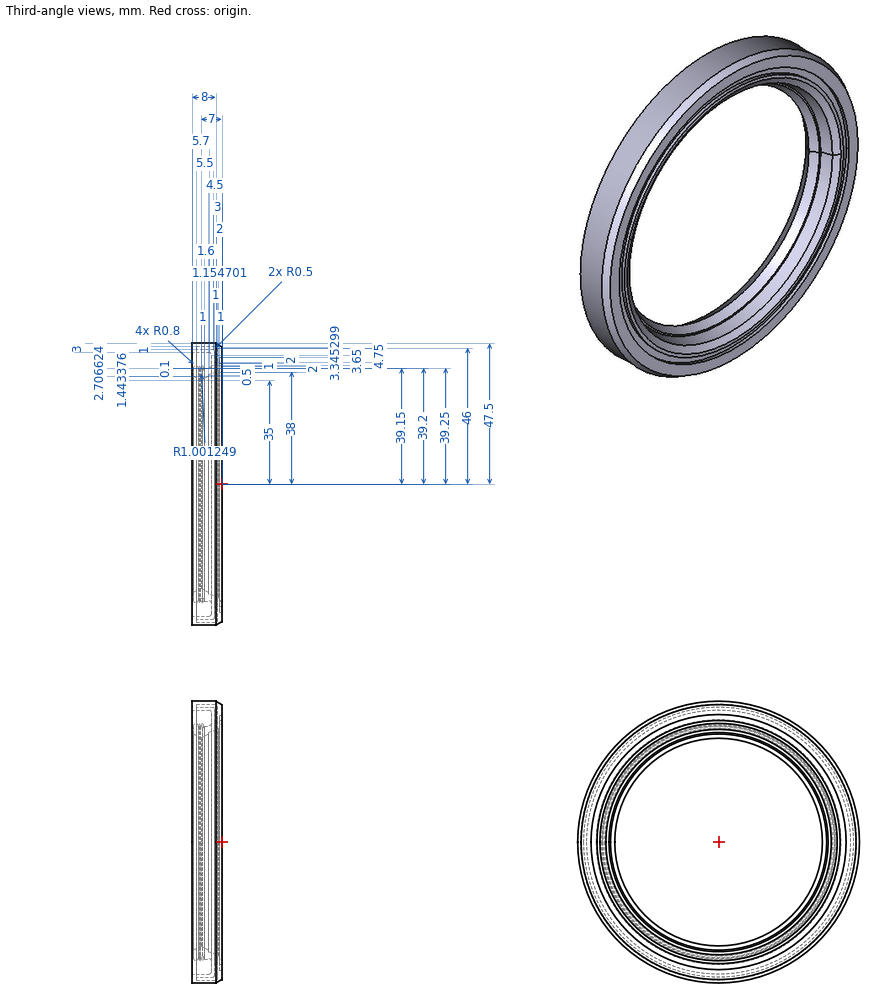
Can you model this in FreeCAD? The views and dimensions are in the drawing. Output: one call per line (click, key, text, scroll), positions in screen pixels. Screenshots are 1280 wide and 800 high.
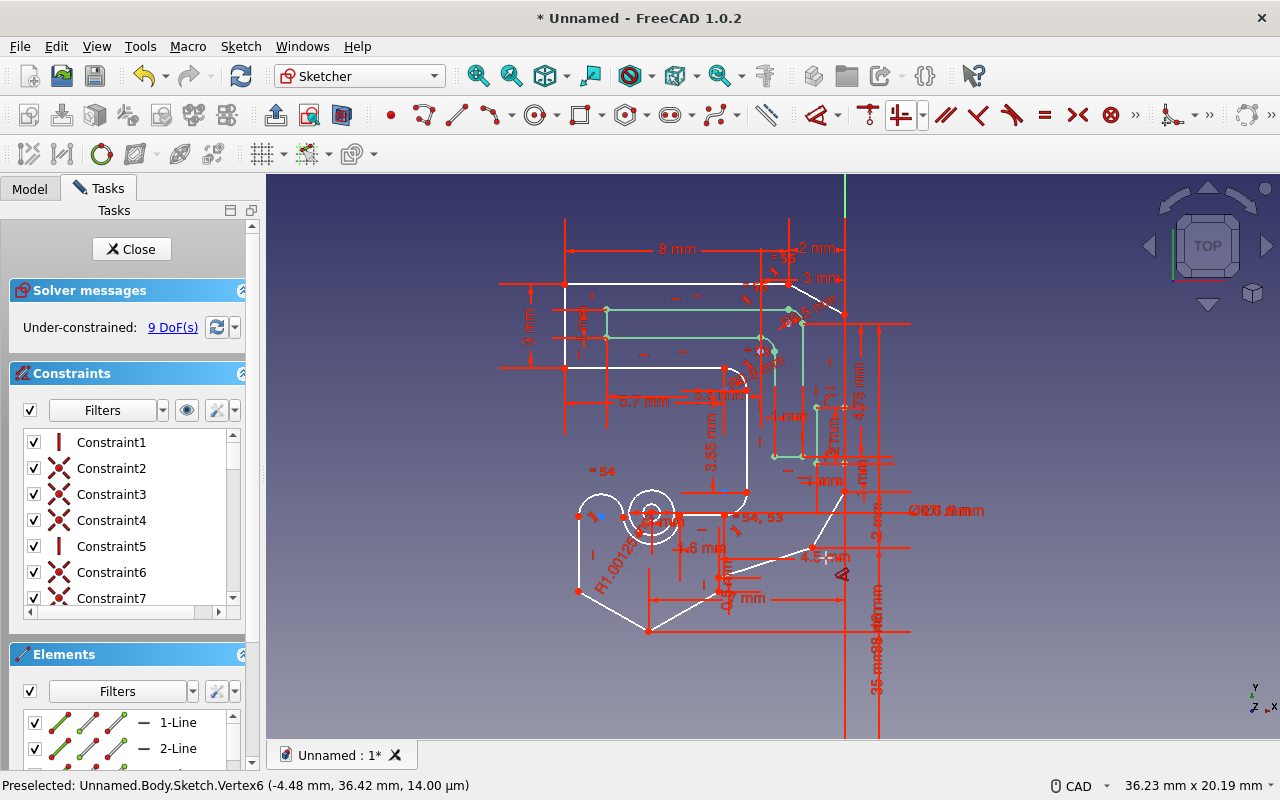
scroll(624, 517, up, 14)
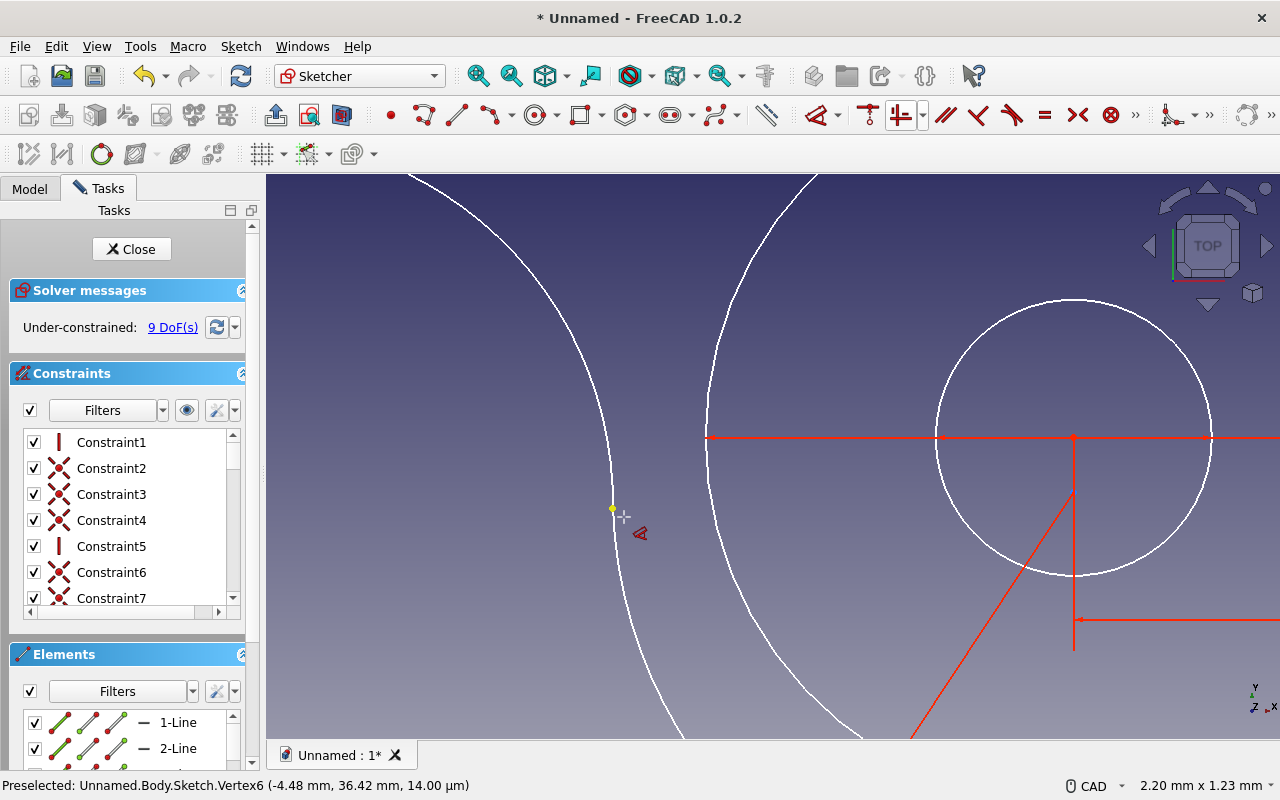
click(613, 508)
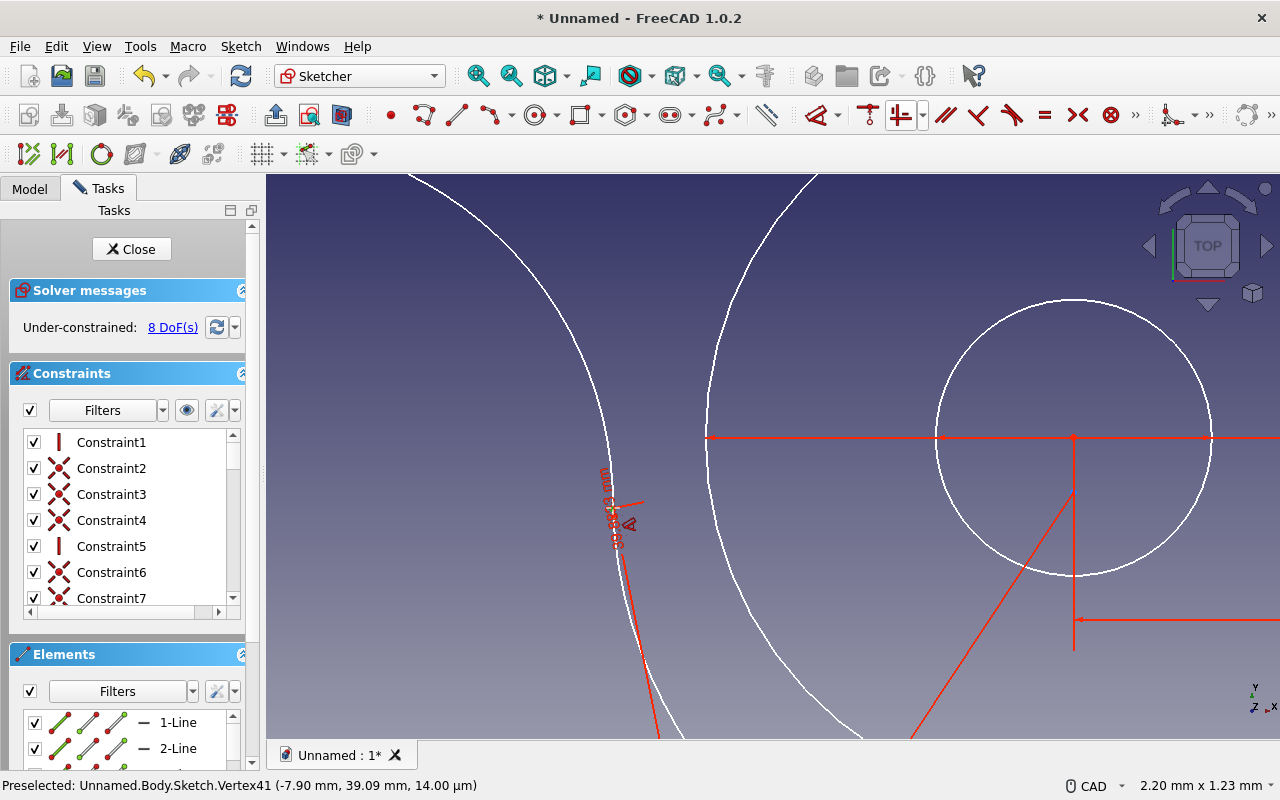
click(1074, 438)
click(579, 473)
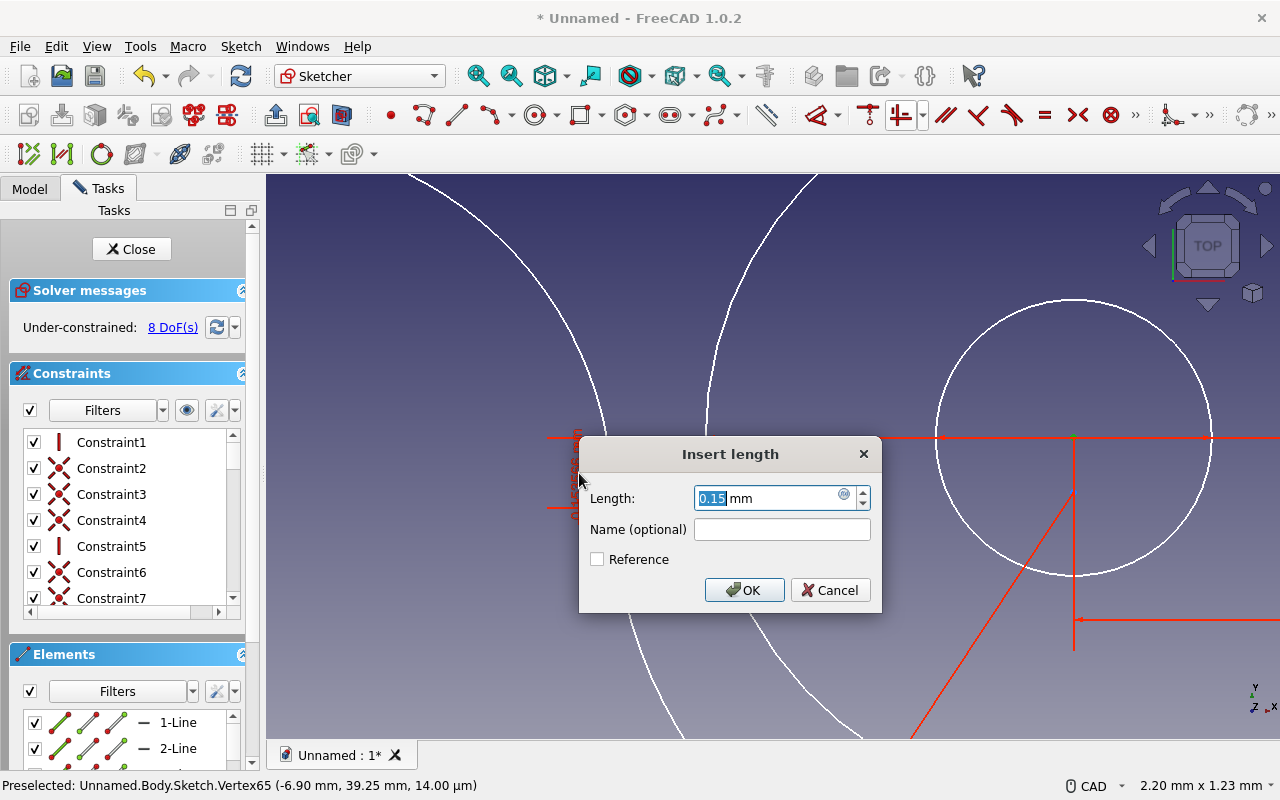
text(0.1)
key(Return)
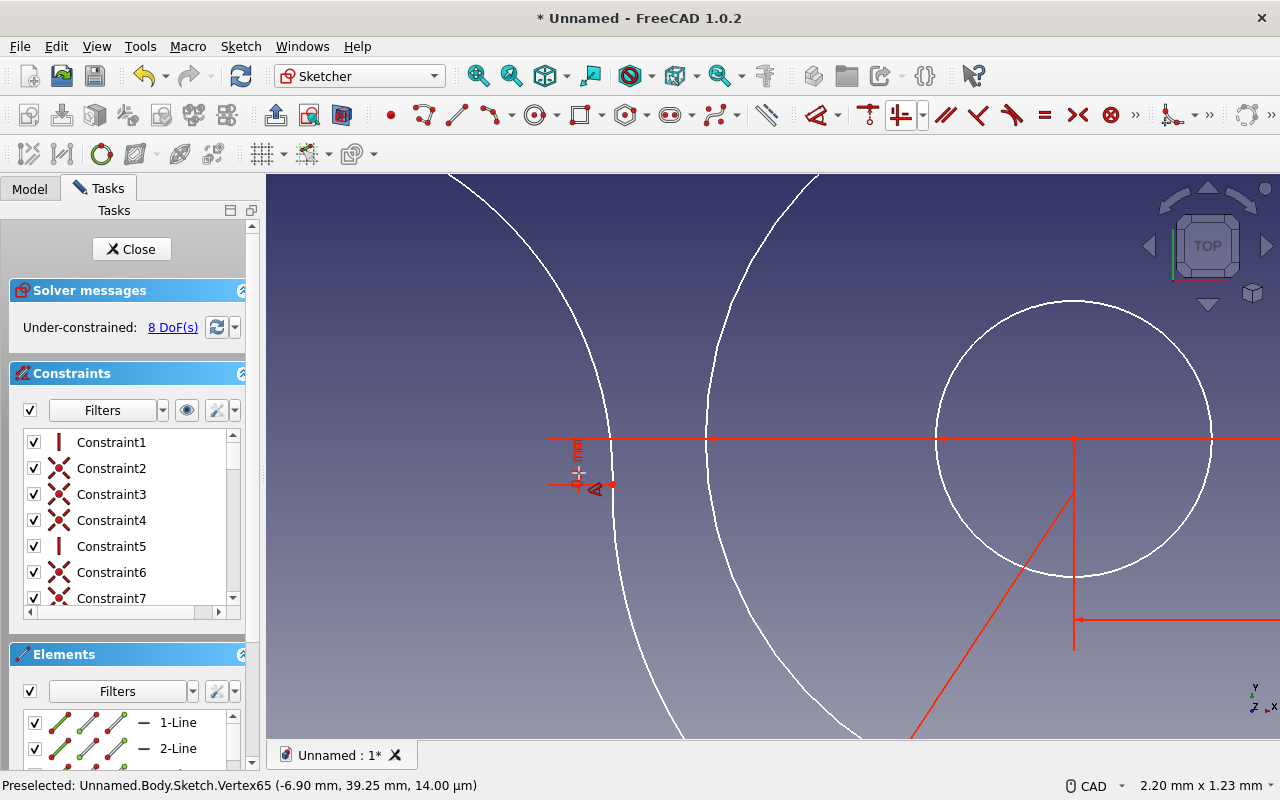
scroll(624, 517, down, 14)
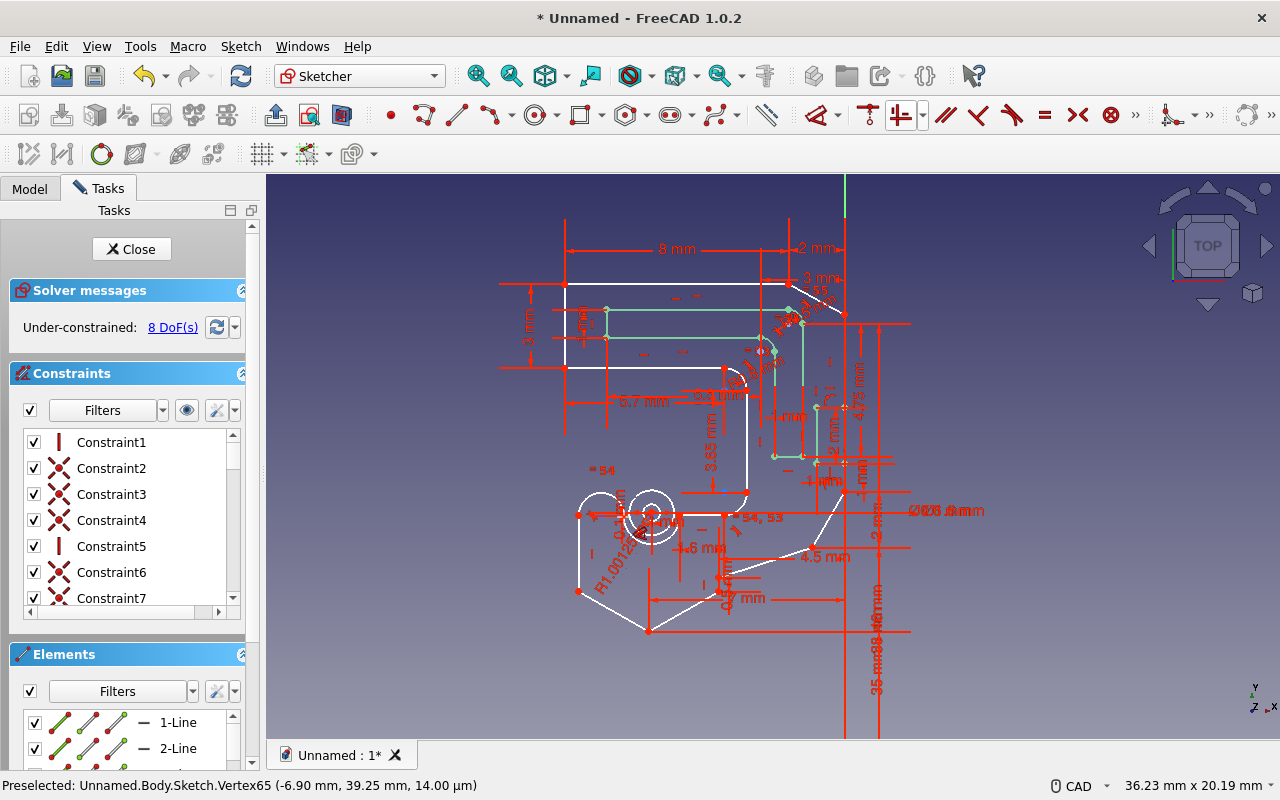
click(789, 284)
click(879, 348)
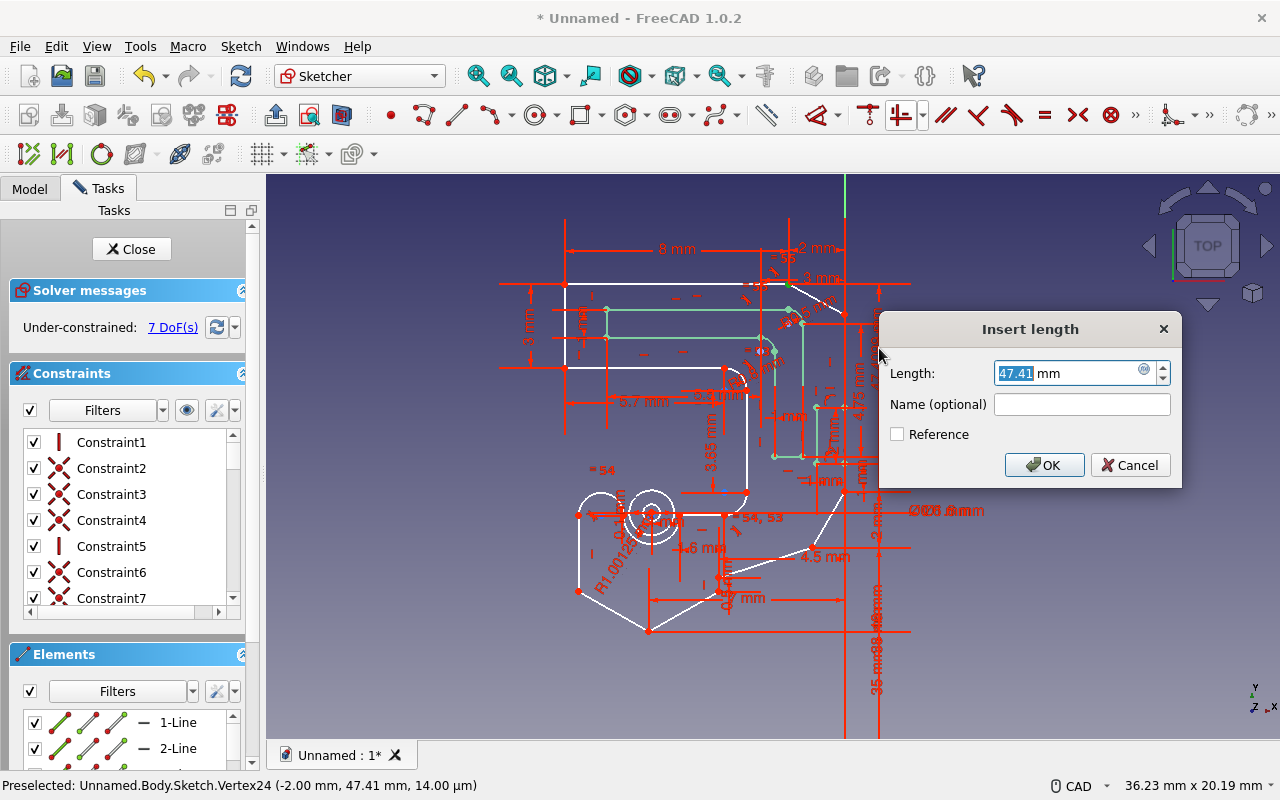
text(47.5)
key(Return)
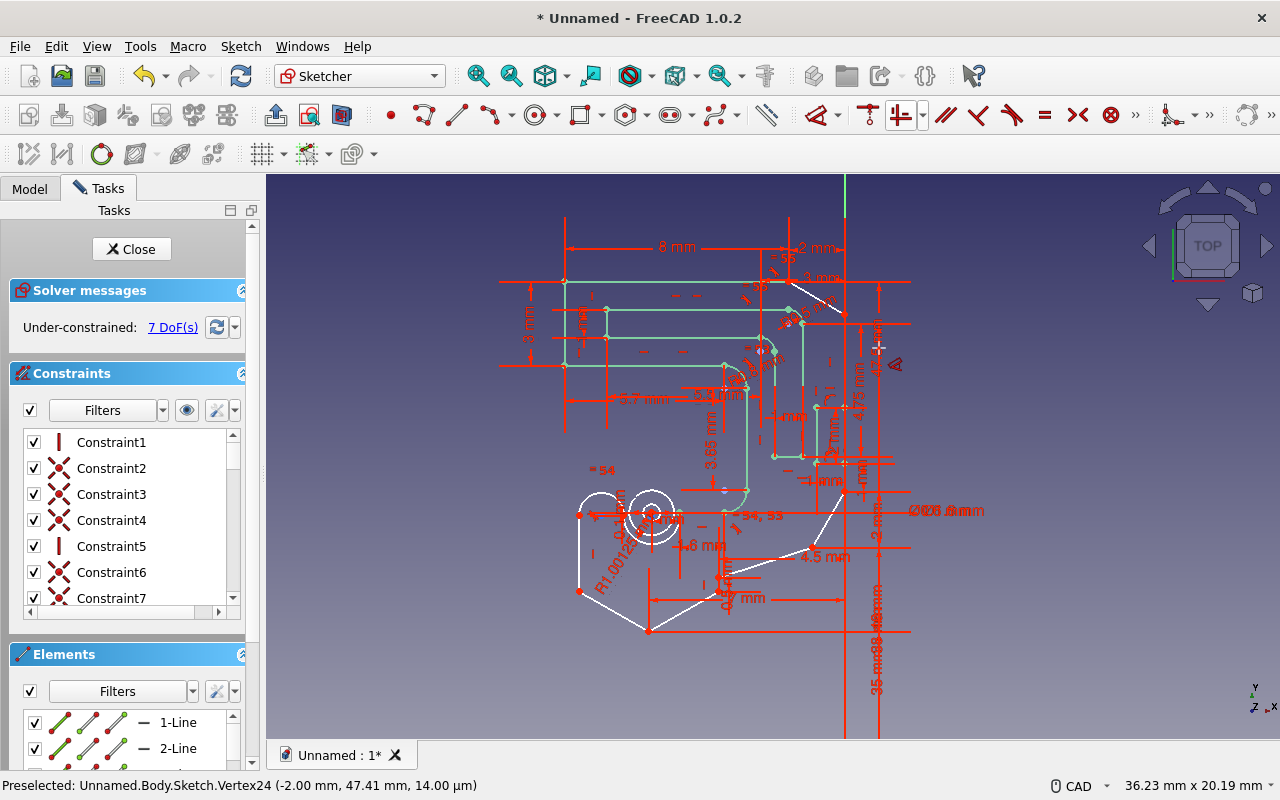
scroll(652, 516, up, 7)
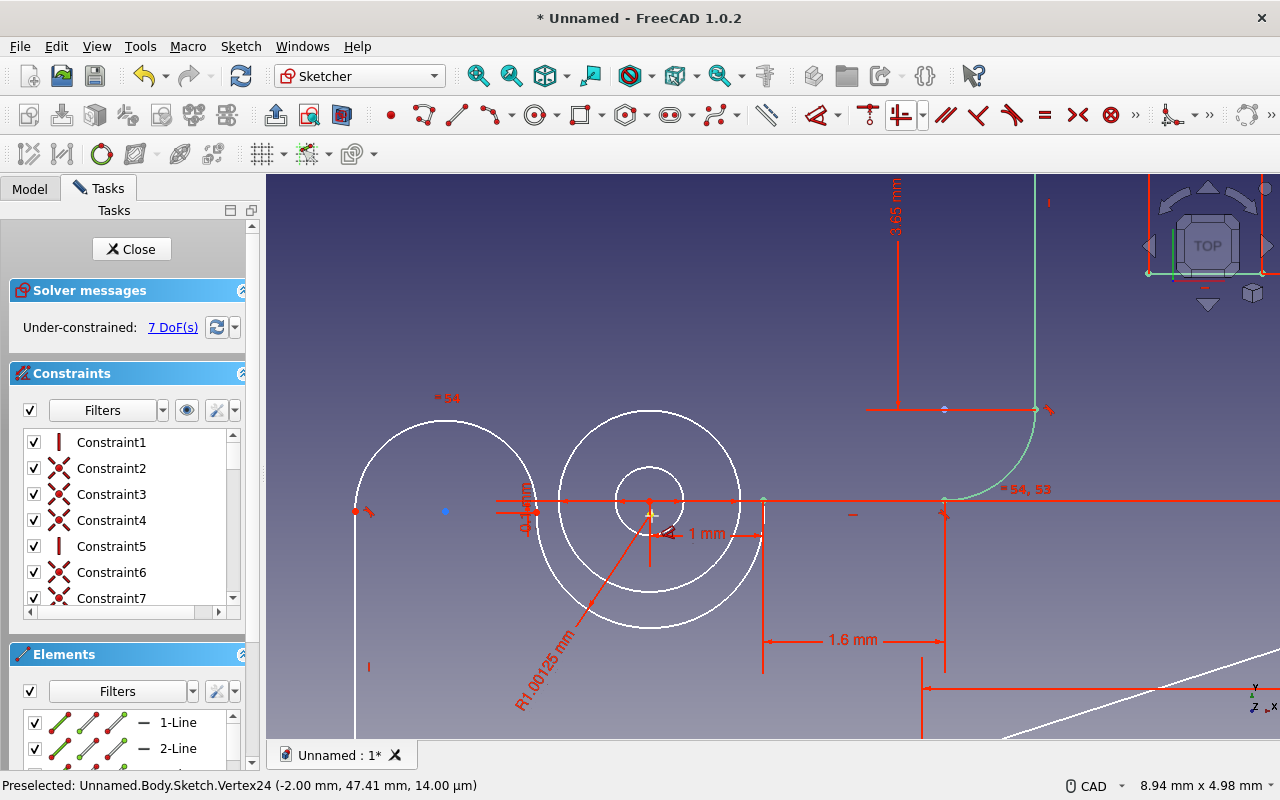
click(650, 514)
click(616, 568)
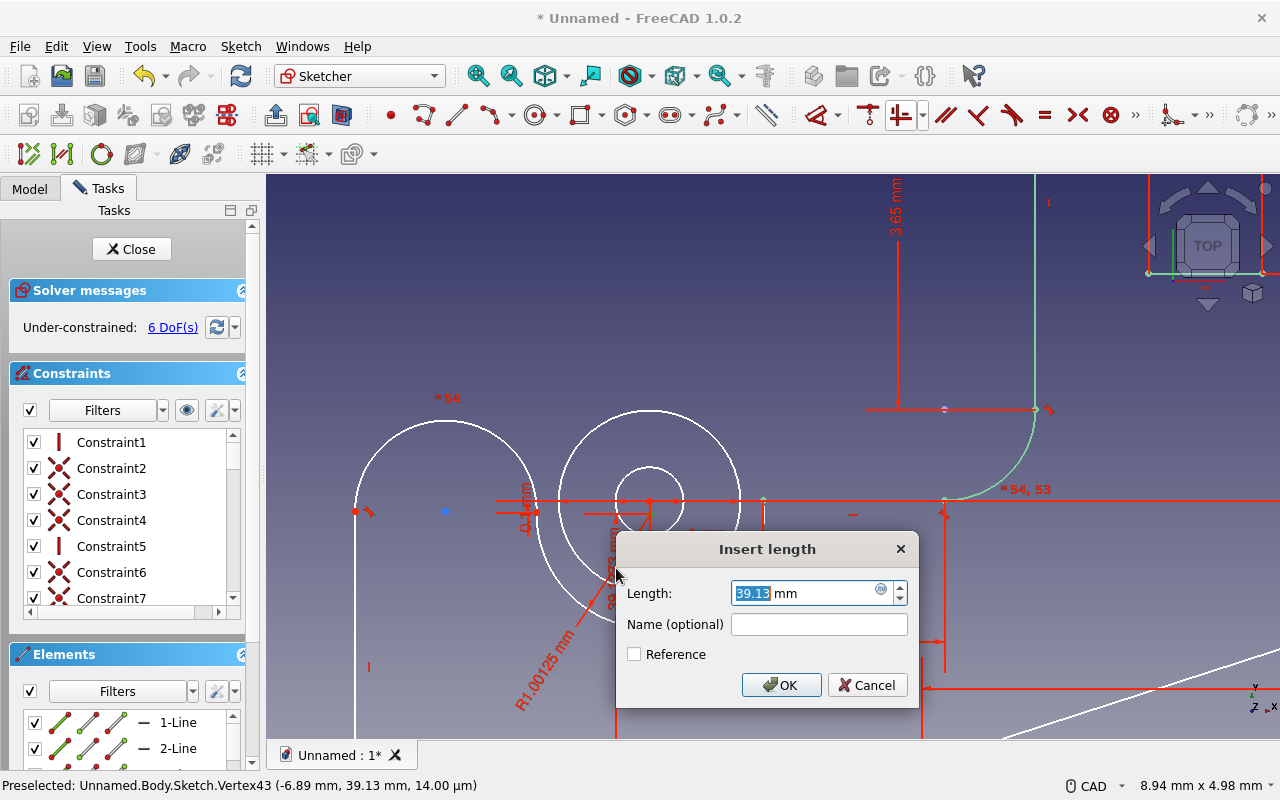
text(39.2)
key(Return)